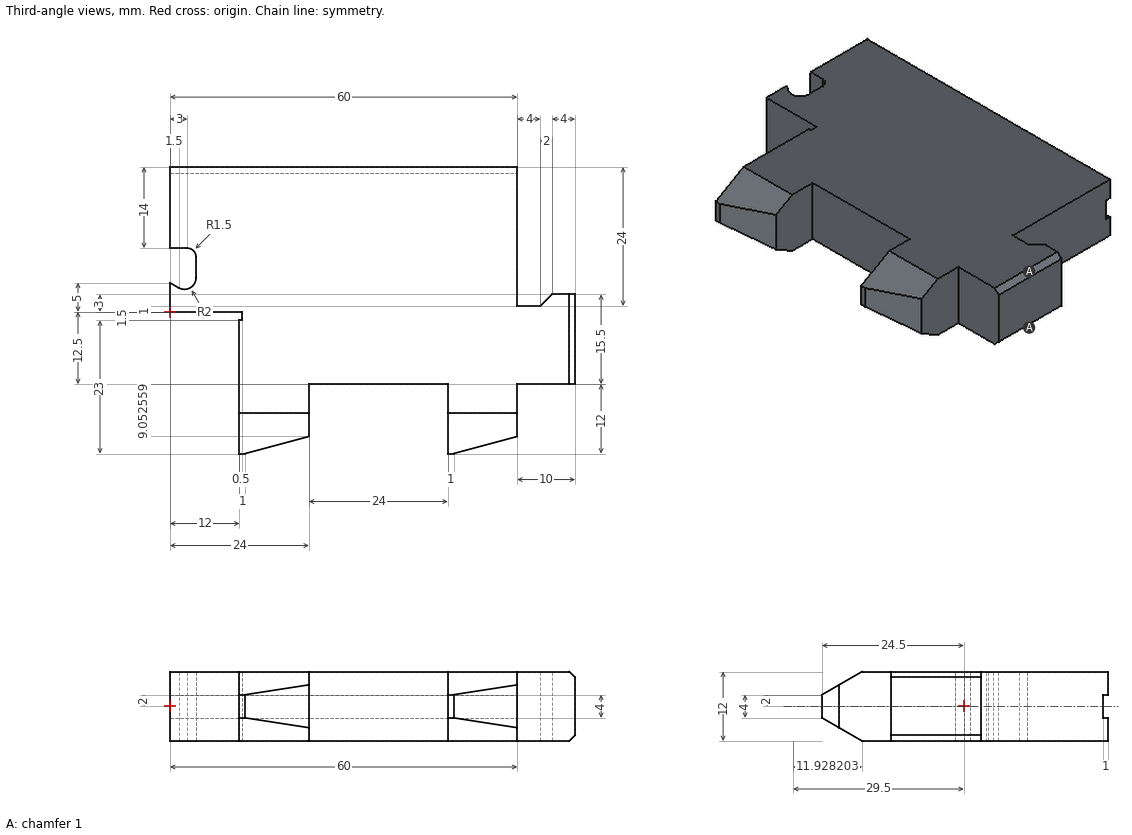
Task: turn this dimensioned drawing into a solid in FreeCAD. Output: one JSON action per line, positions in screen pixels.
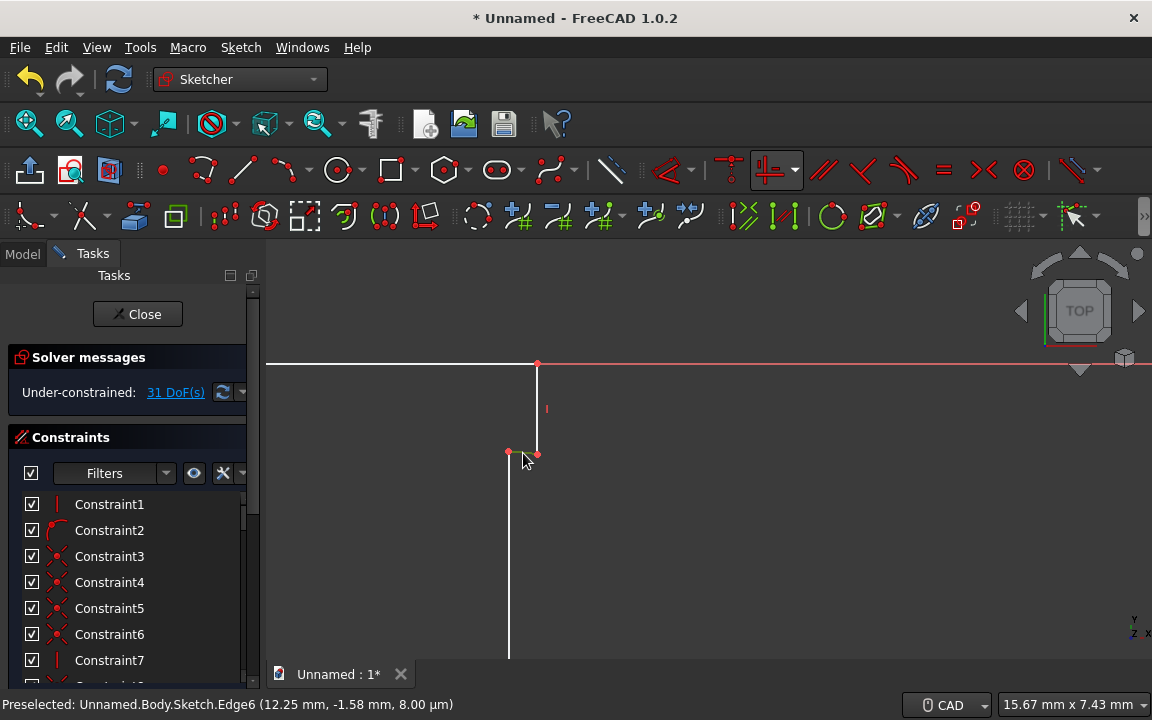
{"action": "key", "text": "h"}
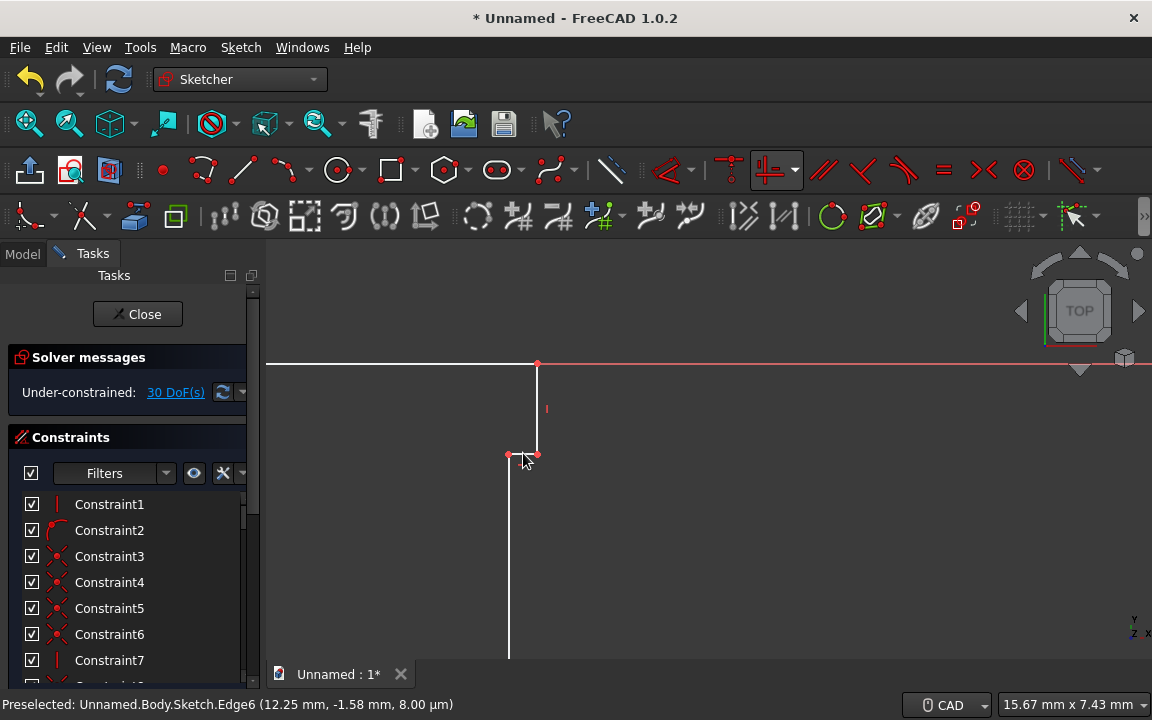
{"action": "scroll", "coordinate": [524, 459], "scroll_direction": "down", "scroll_amount": 12}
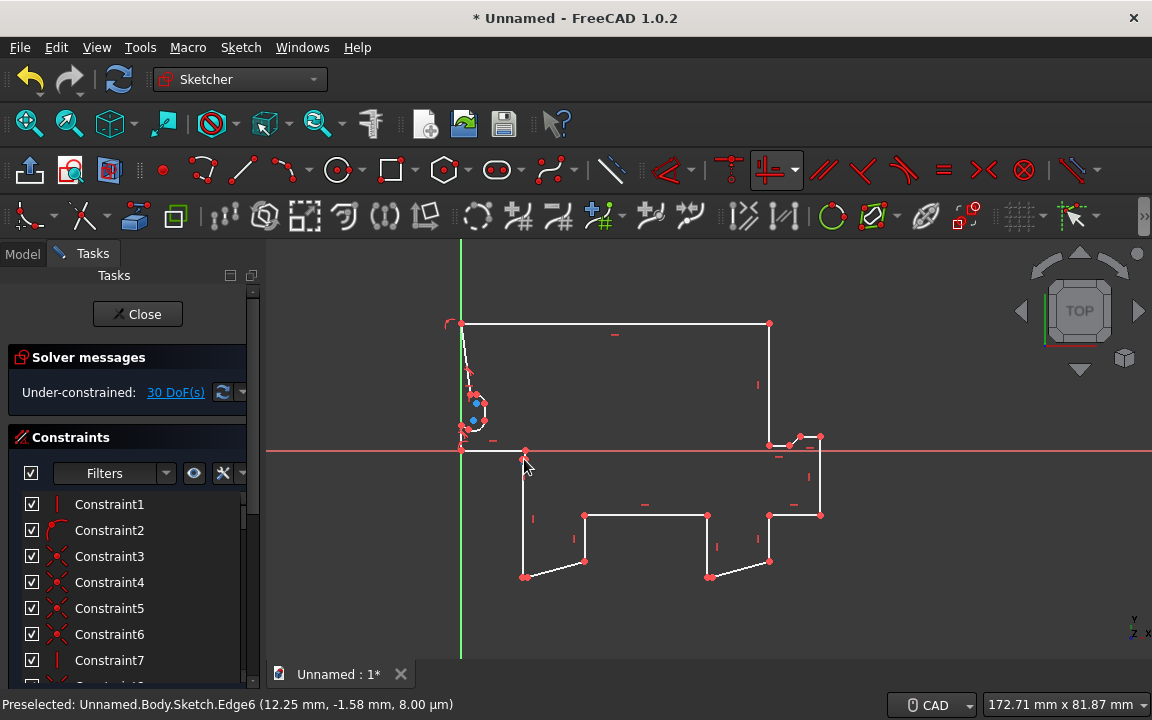
{"action": "scroll", "coordinate": [524, 578], "scroll_direction": "up", "scroll_amount": 12}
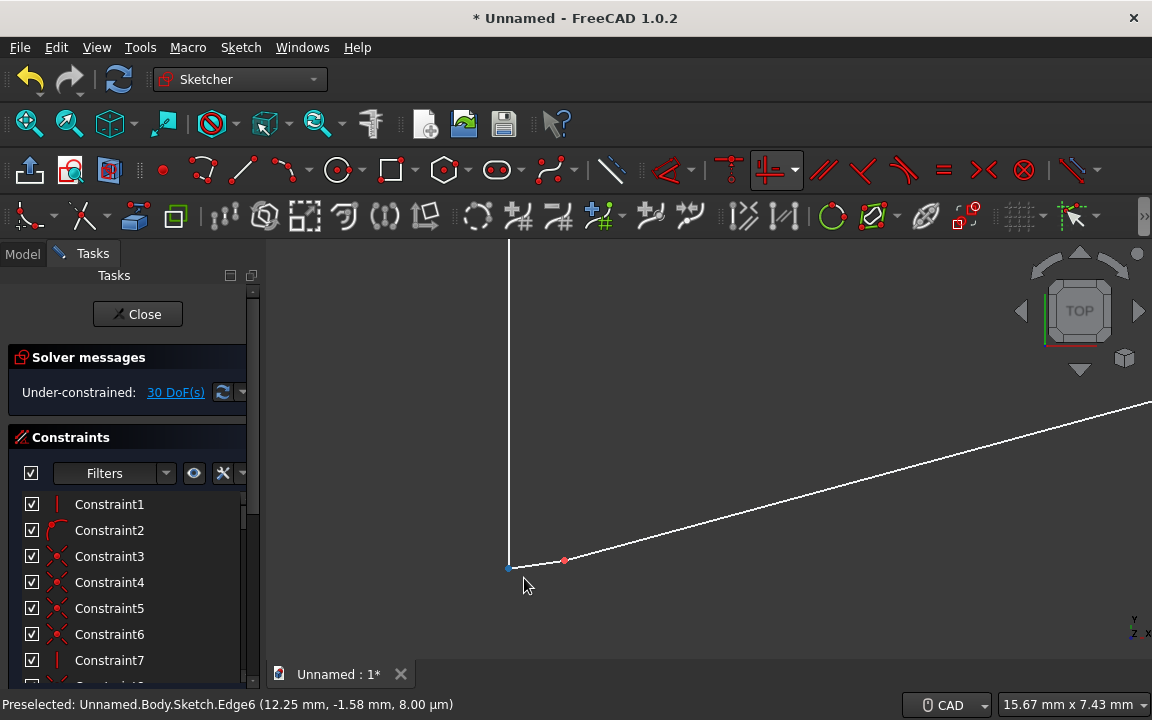
{"action": "left_click", "coordinate": [525, 566]}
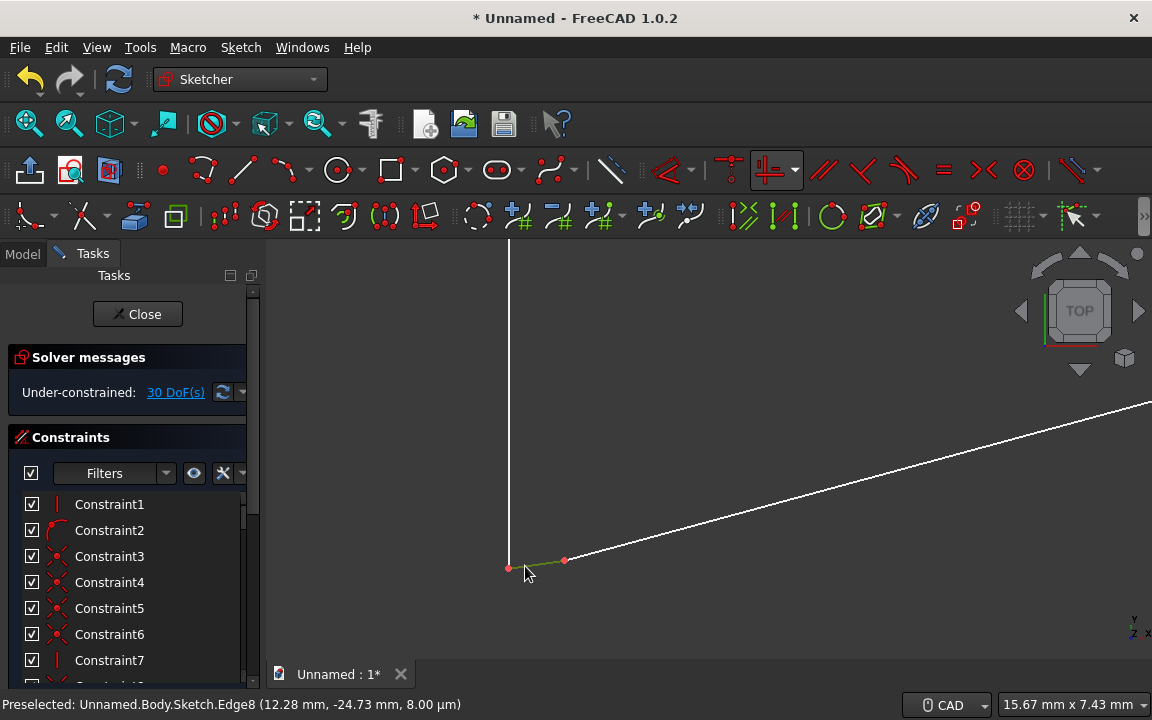
{"action": "left_click", "coordinate": [798, 170]}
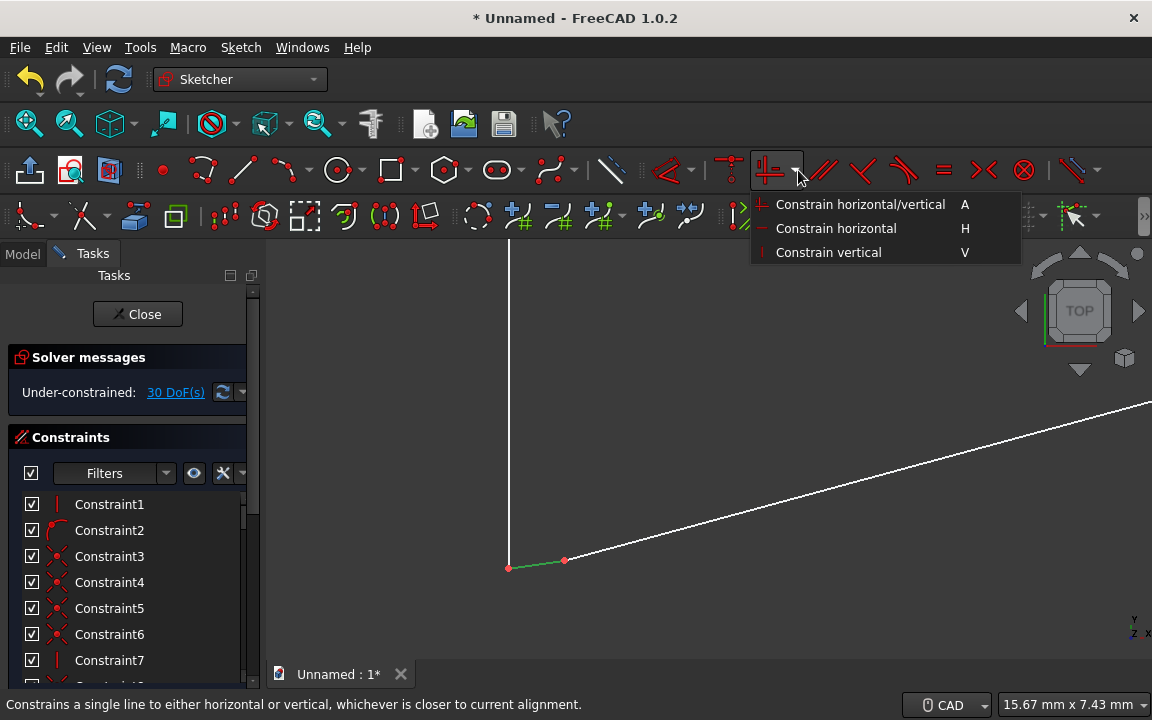
{"action": "left_click", "coordinate": [886, 228]}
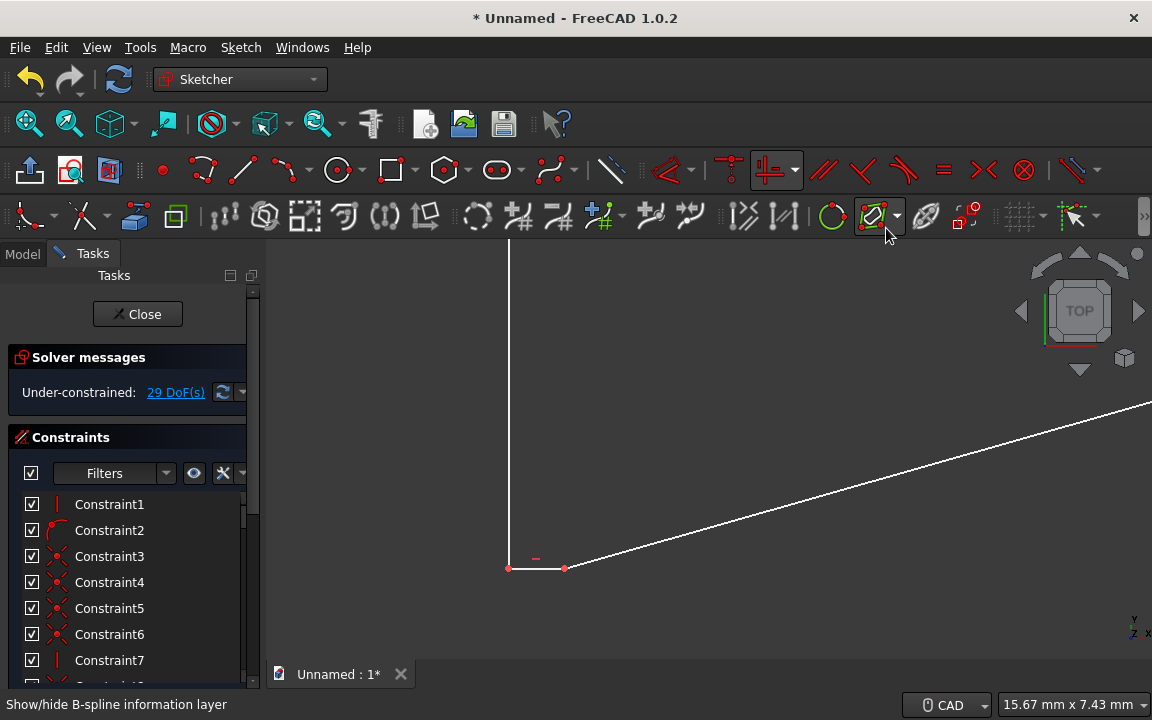
{"action": "scroll", "coordinate": [524, 578], "scroll_direction": "down", "scroll_amount": 12}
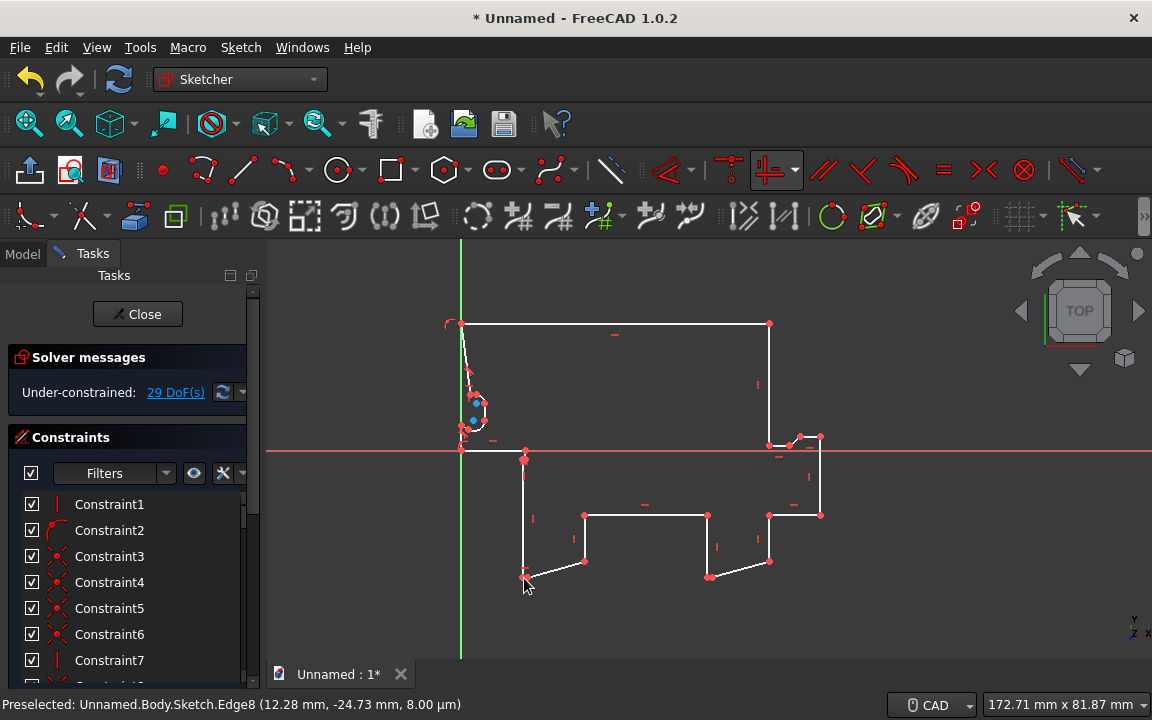
{"action": "scroll", "coordinate": [709, 578], "scroll_direction": "up", "scroll_amount": 11}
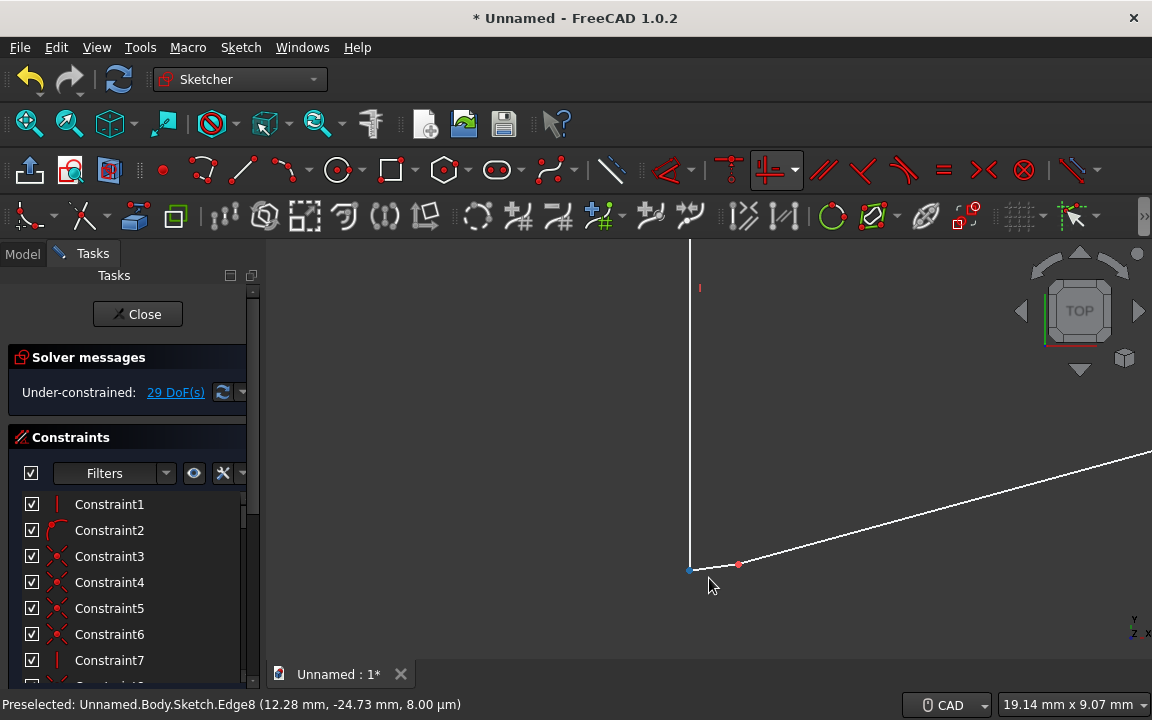
{"action": "left_click", "coordinate": [704, 569]}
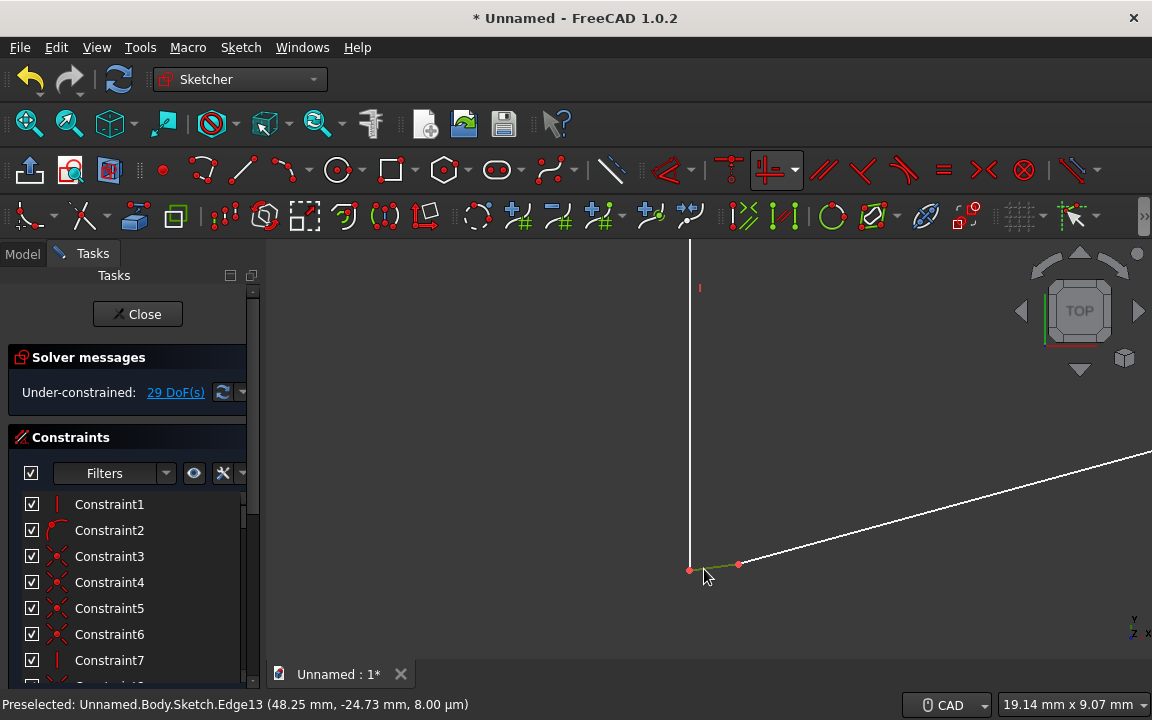
{"action": "left_click", "coordinate": [798, 170]}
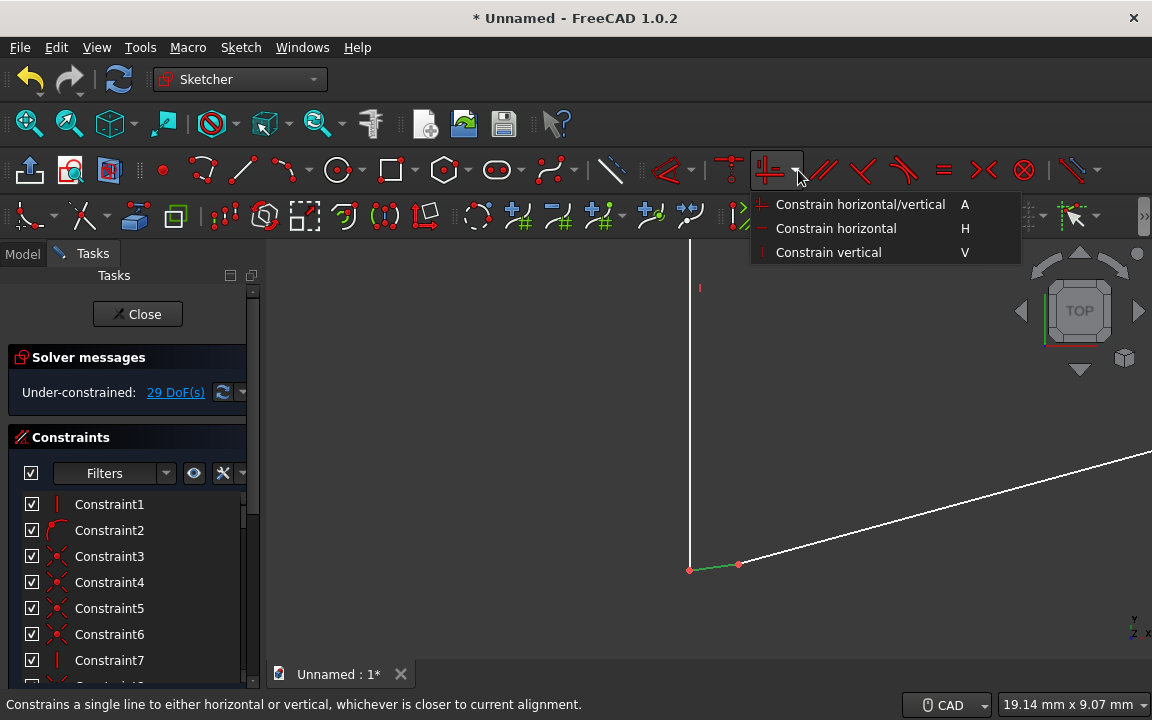
{"action": "left_click", "coordinate": [886, 228]}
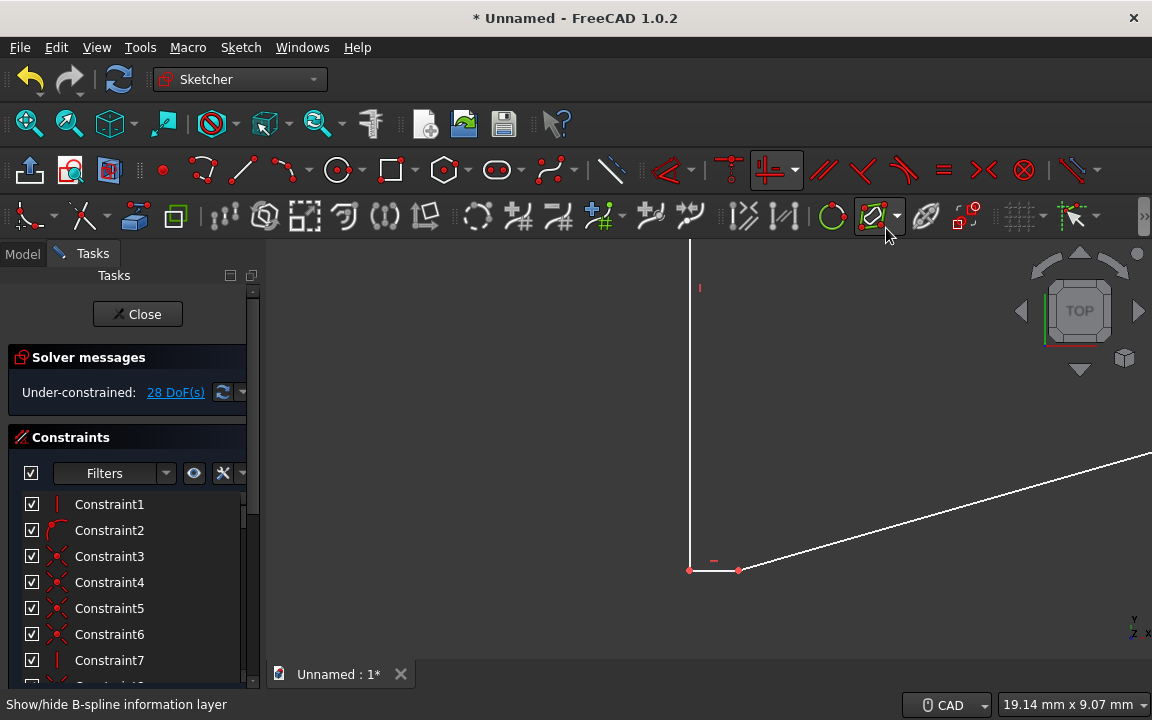
{"action": "scroll", "coordinate": [709, 578], "scroll_direction": "down", "scroll_amount": 11}